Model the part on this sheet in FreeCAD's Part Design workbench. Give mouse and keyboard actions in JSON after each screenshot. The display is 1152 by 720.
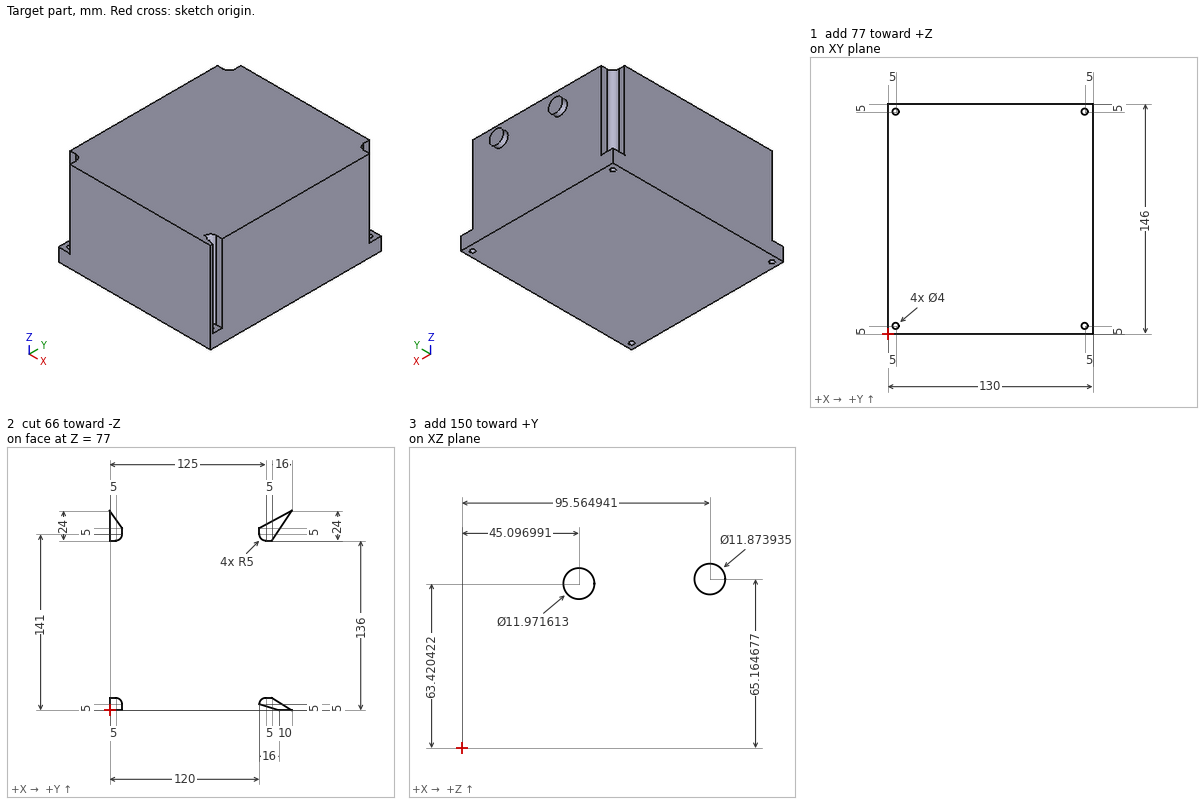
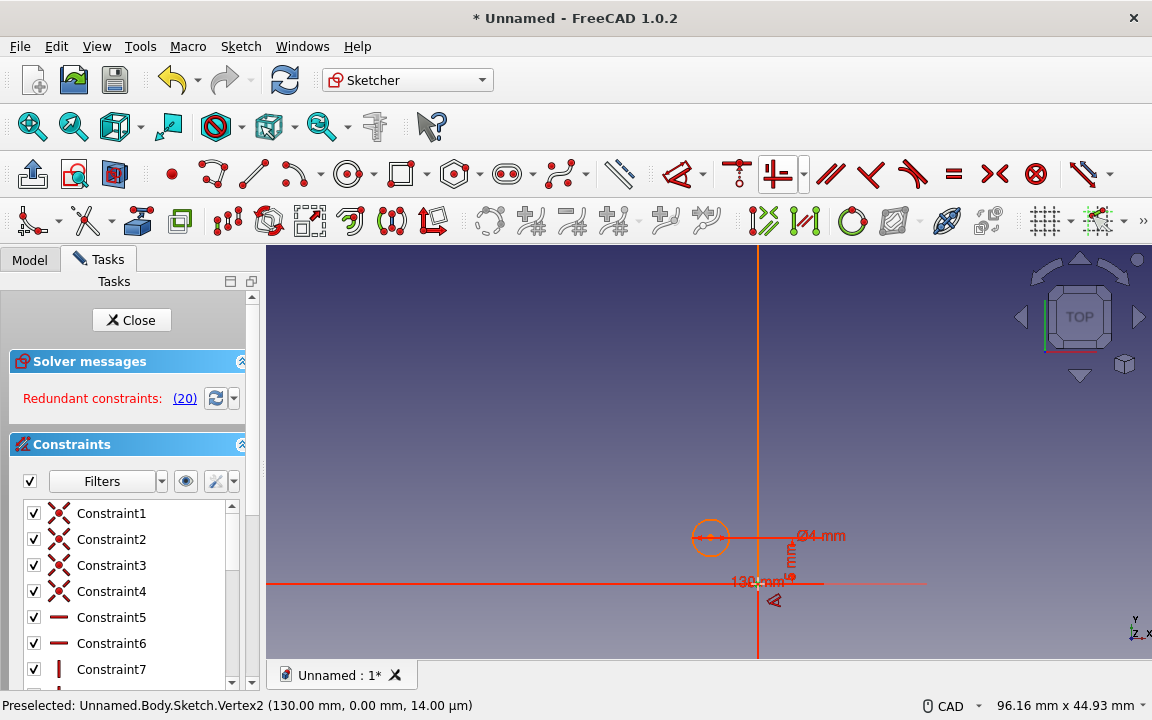
{"action": "left_click", "coordinate": [711, 538]}
{"action": "left_click", "coordinate": [734, 618]}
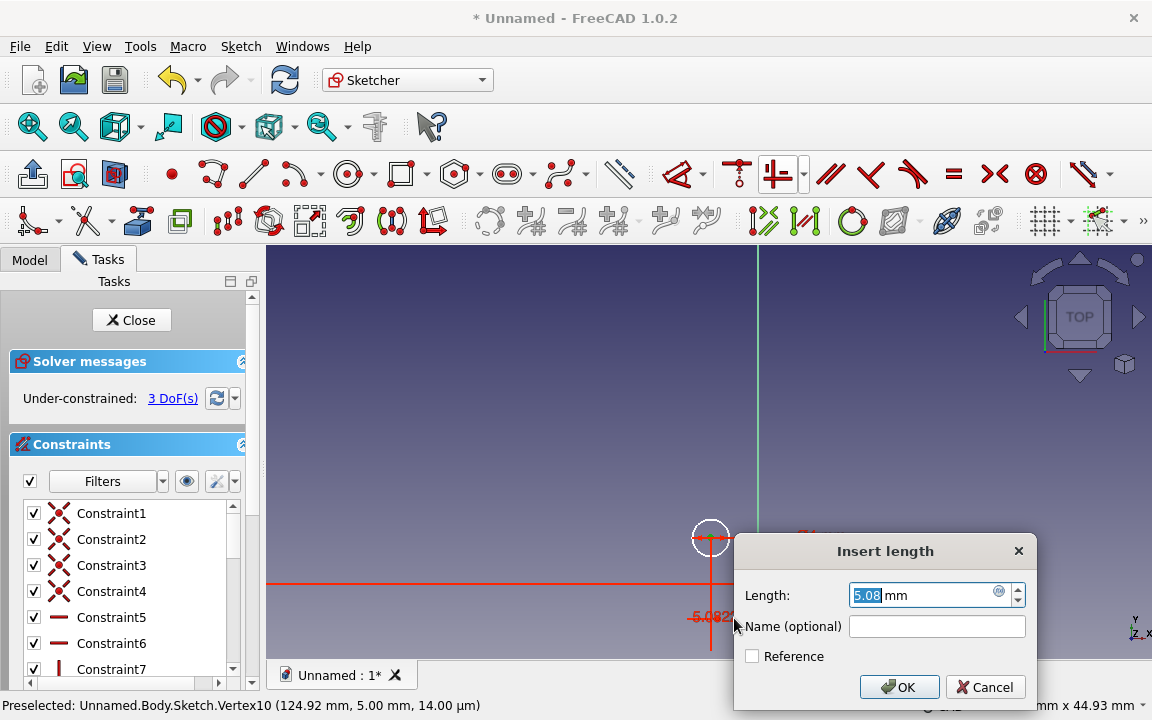
{"action": "type", "text": "5"}
{"action": "key", "text": "Return"}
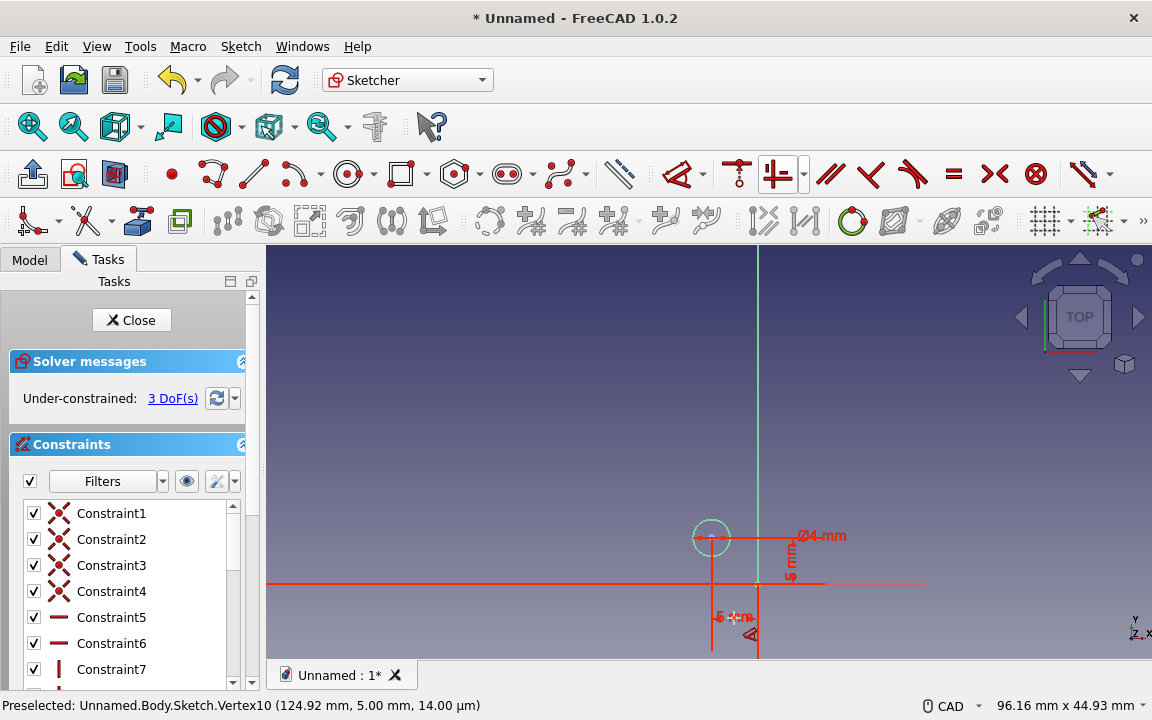
{"action": "scroll", "coordinate": [762, 589], "scroll_direction": "down", "scroll_amount": 8}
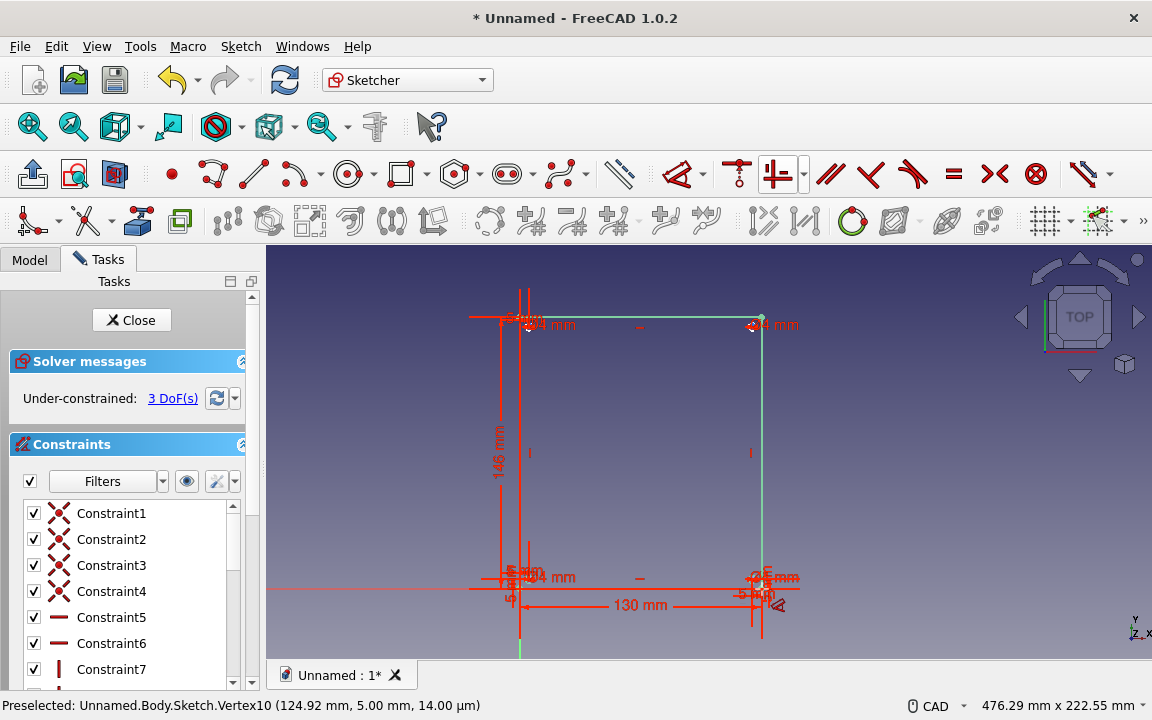
{"action": "scroll", "coordinate": [520, 317], "scroll_direction": "up", "scroll_amount": 8}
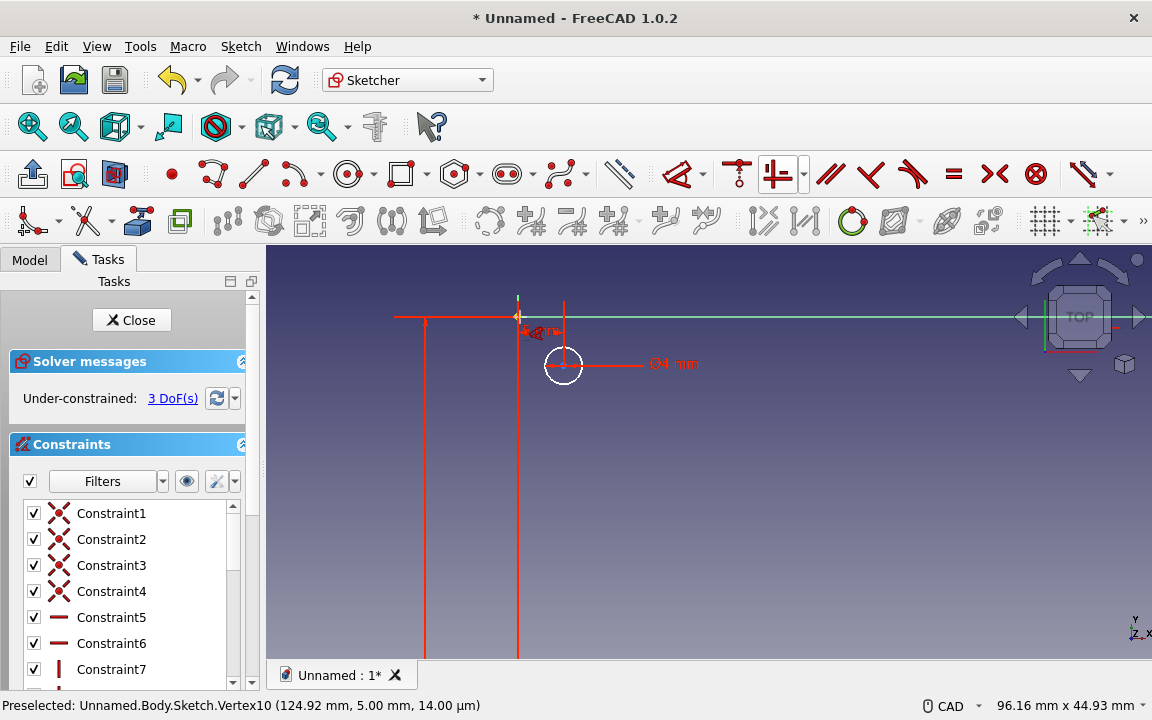
{"action": "left_click", "coordinate": [518, 317]}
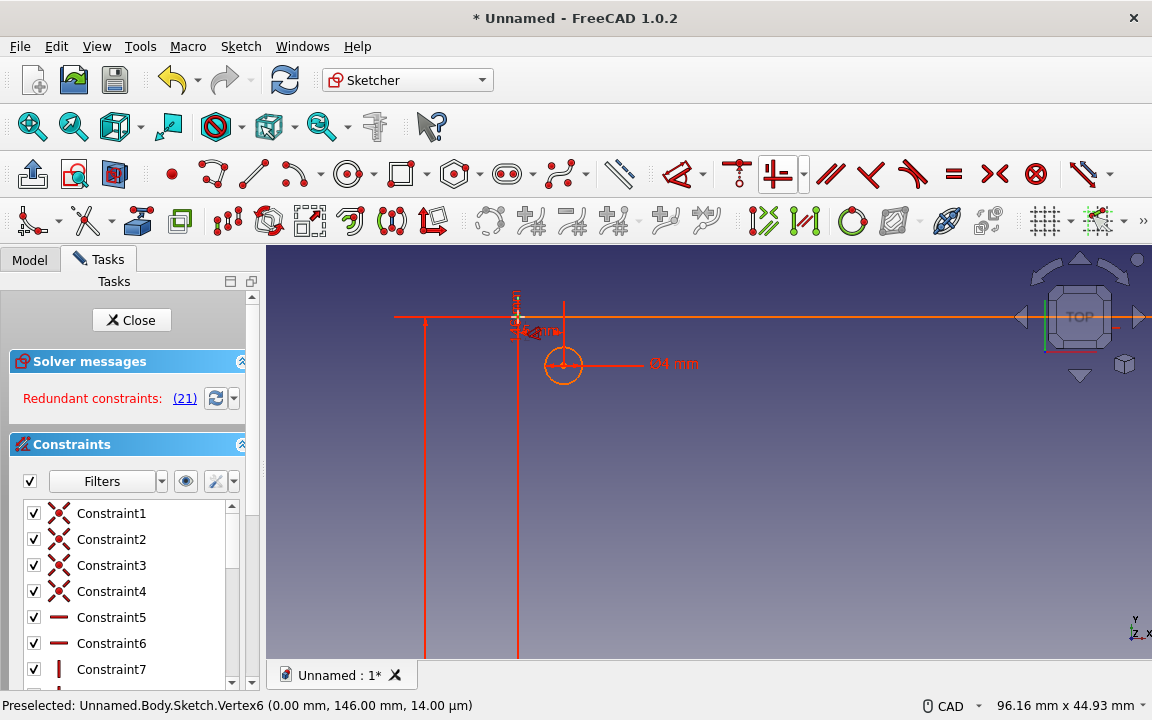
{"action": "left_click", "coordinate": [564, 366]}
{"action": "left_click", "coordinate": [484, 353]}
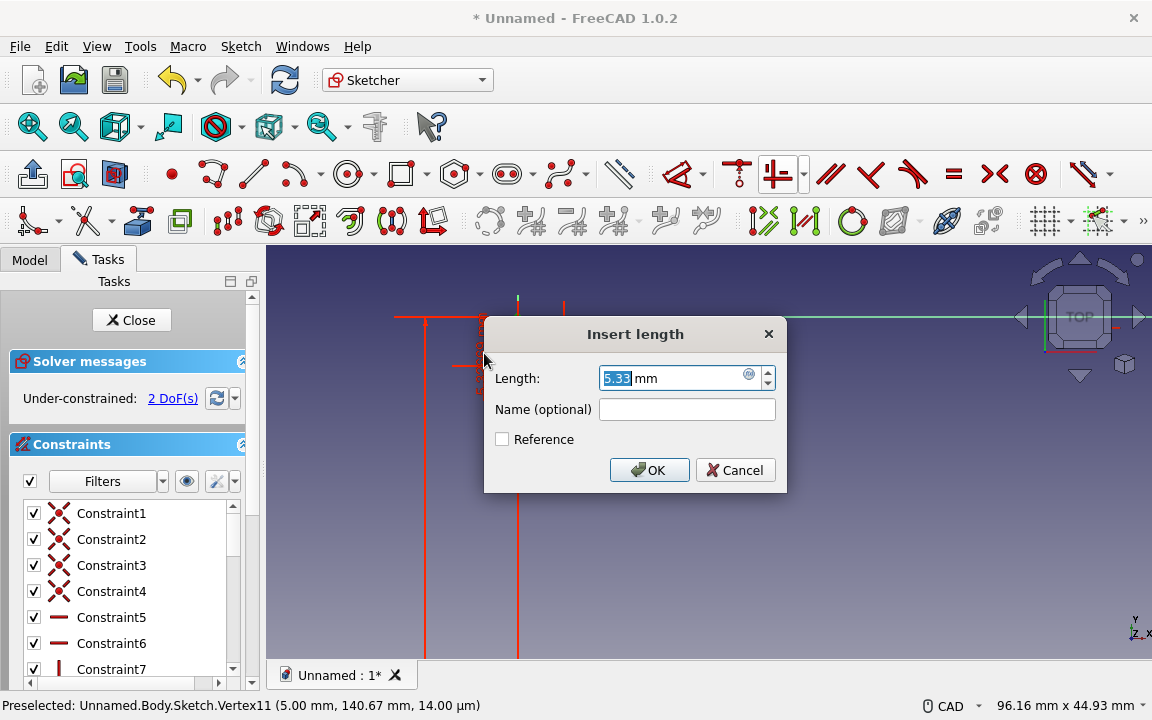
{"action": "type", "text": "5"}
{"action": "key", "text": "Return"}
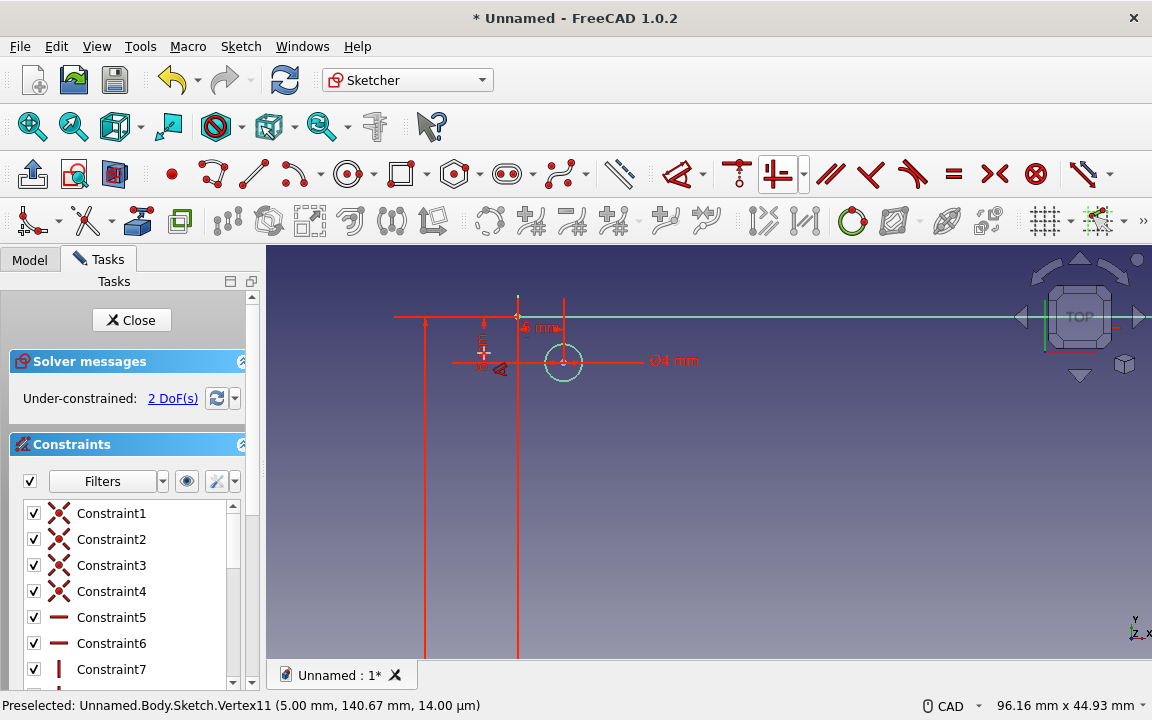
{"action": "scroll", "coordinate": [520, 316], "scroll_direction": "down", "scroll_amount": 8}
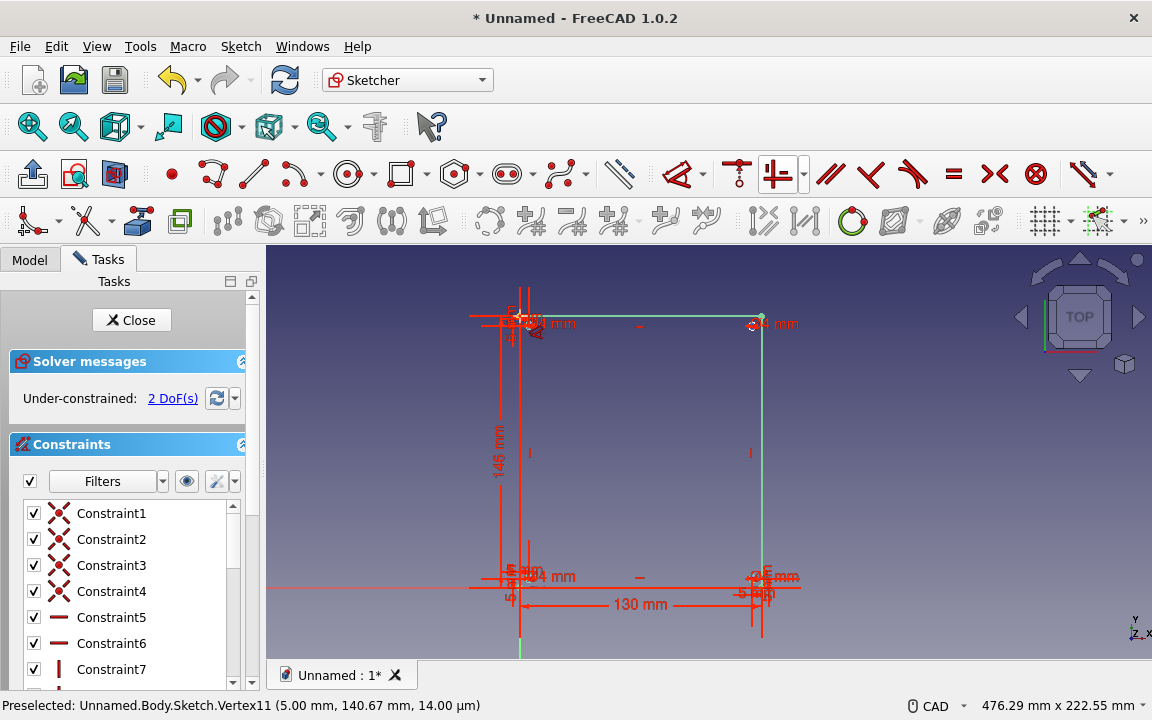
{"action": "scroll", "coordinate": [762, 316], "scroll_direction": "up", "scroll_amount": 8}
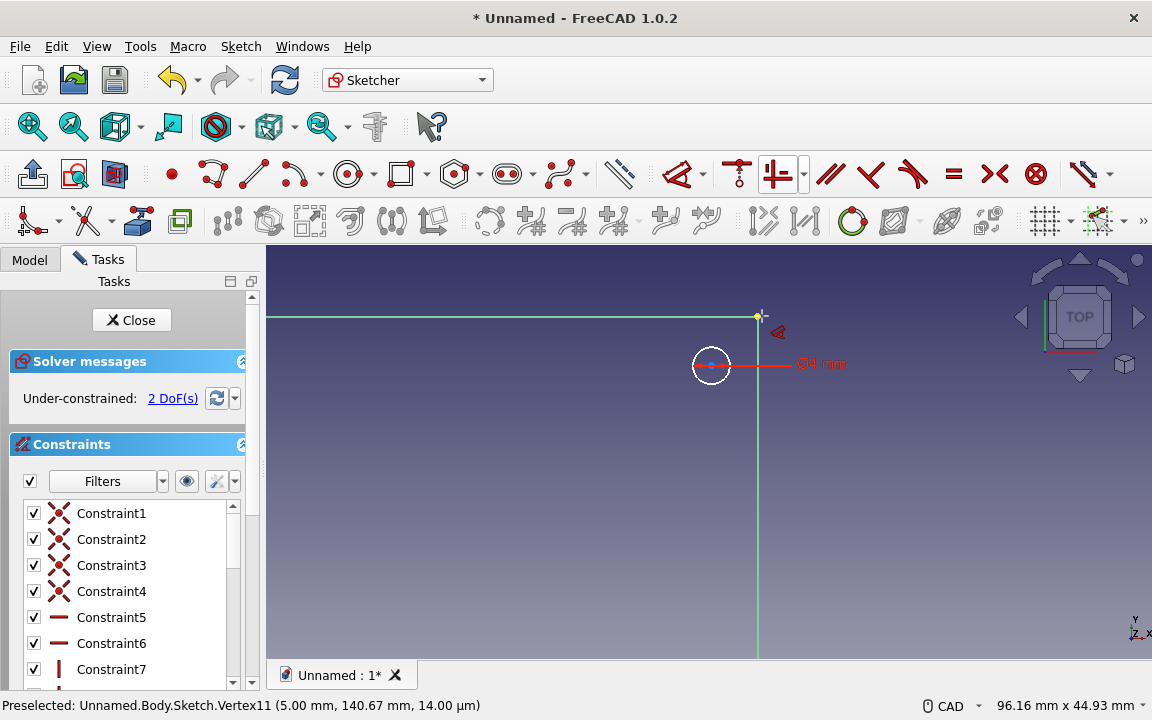
{"action": "left_click", "coordinate": [758, 317]}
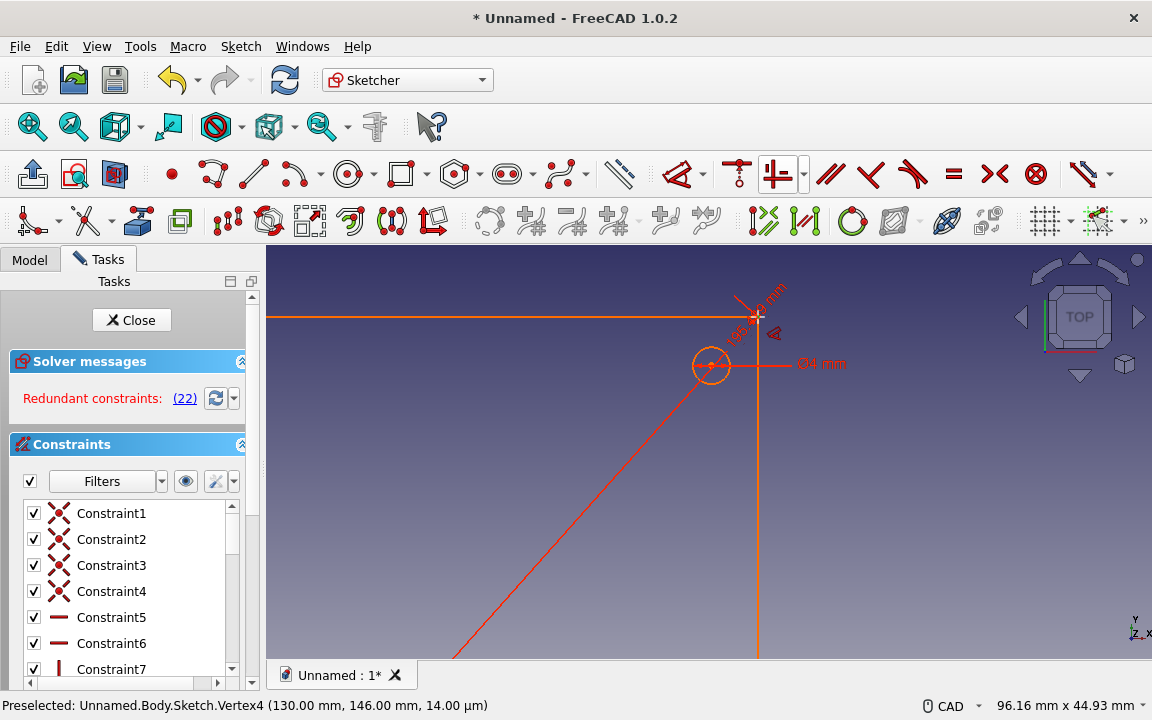
{"action": "left_click", "coordinate": [711, 366]}
{"action": "left_click", "coordinate": [735, 283]}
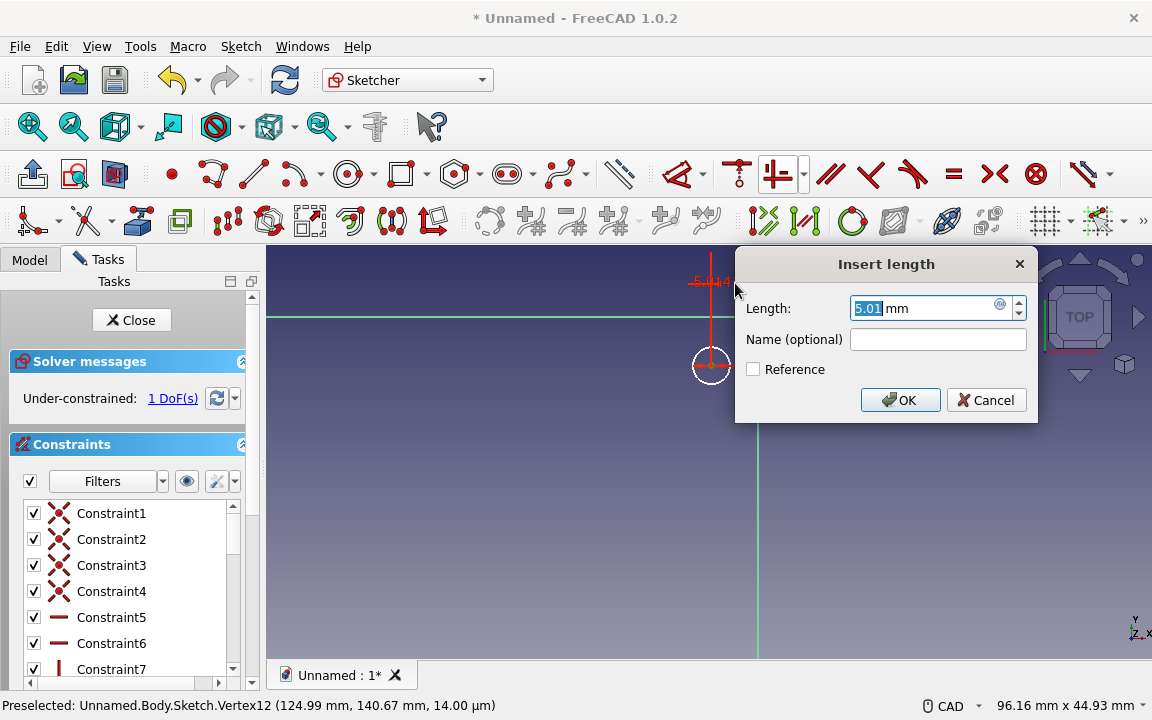
{"action": "type", "text": "5"}
{"action": "key", "text": "Return"}